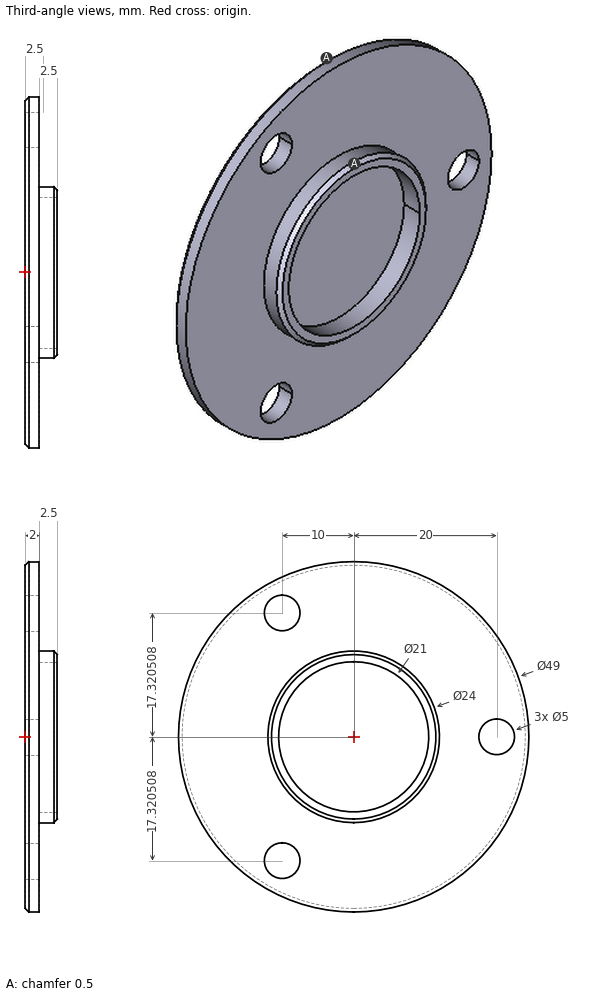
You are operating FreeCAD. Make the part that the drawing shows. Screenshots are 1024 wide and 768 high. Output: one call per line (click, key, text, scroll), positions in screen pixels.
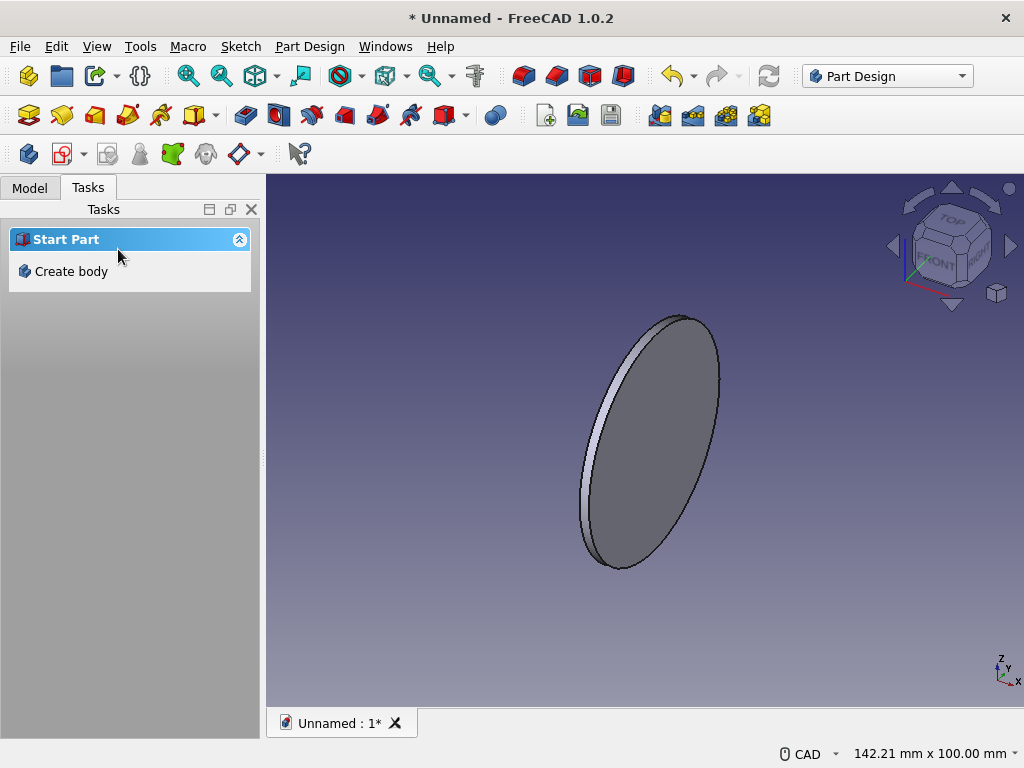
click(654, 443)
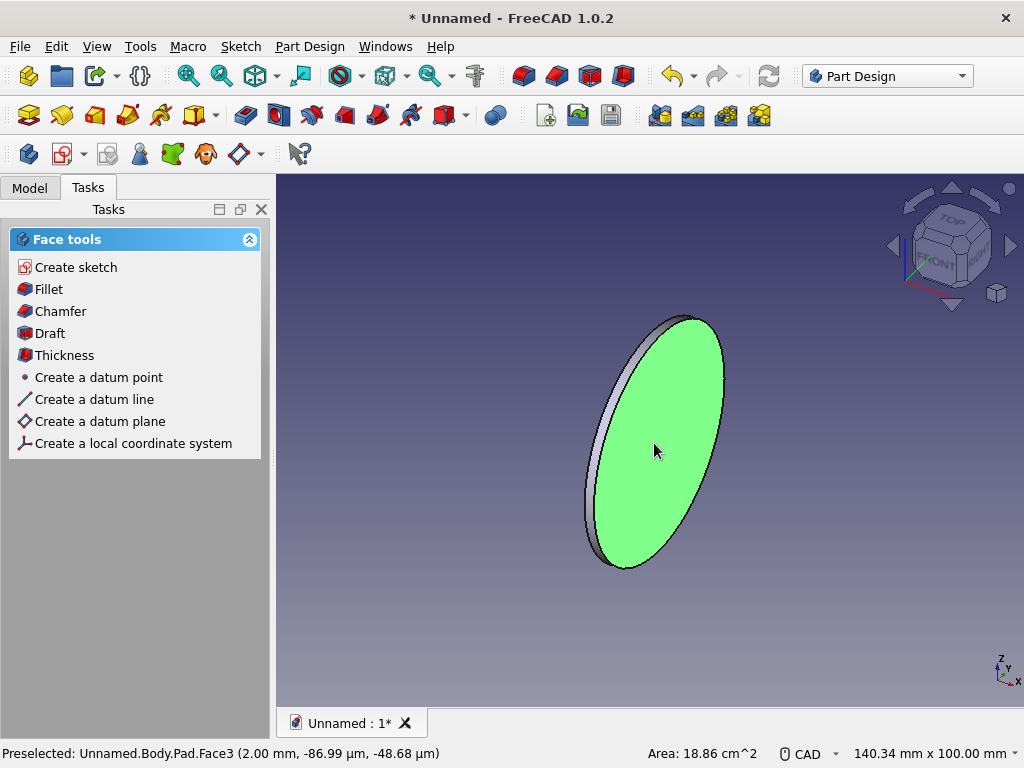
click(62, 154)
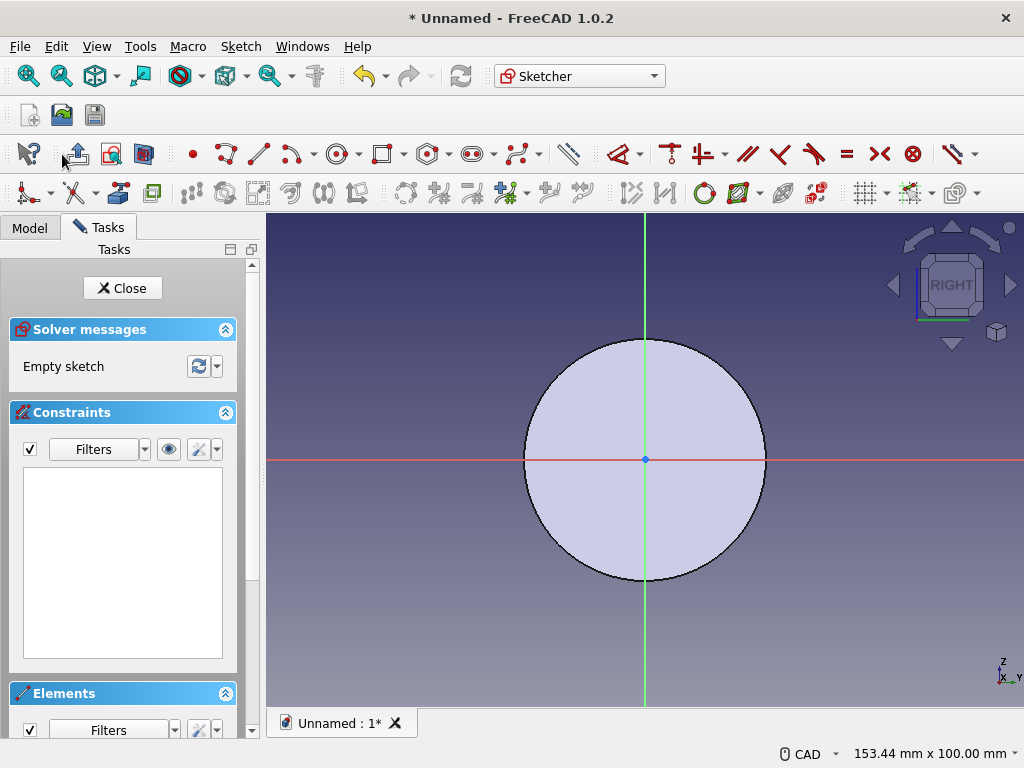
scroll(685, 460, up, 5)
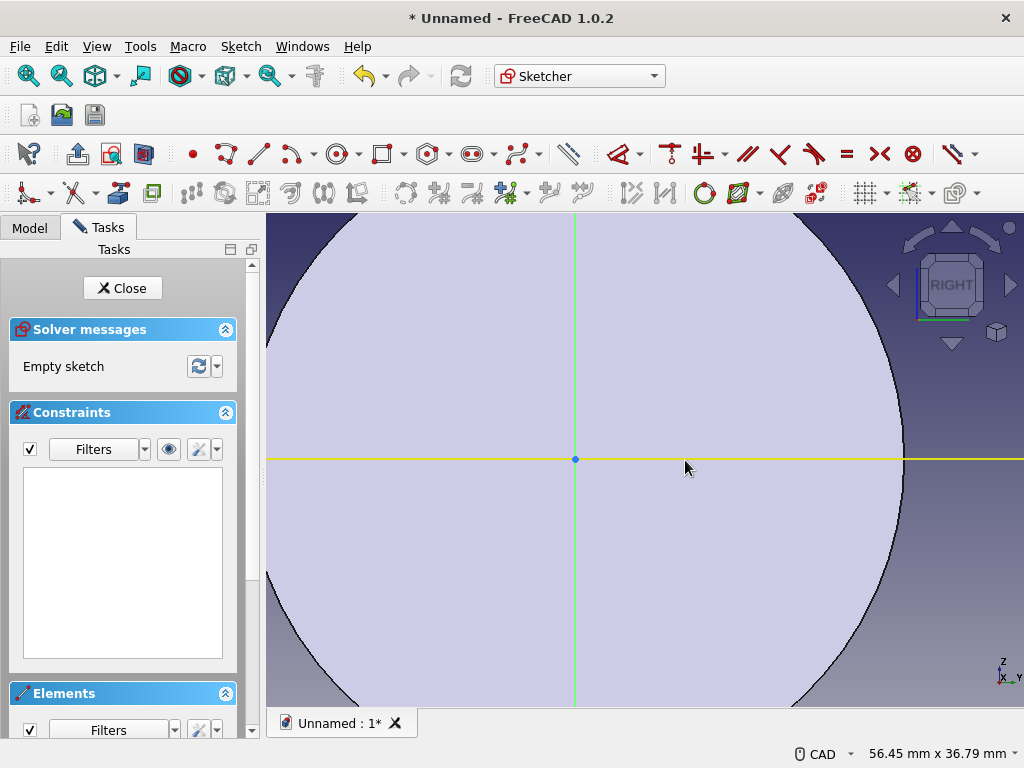
click(336, 154)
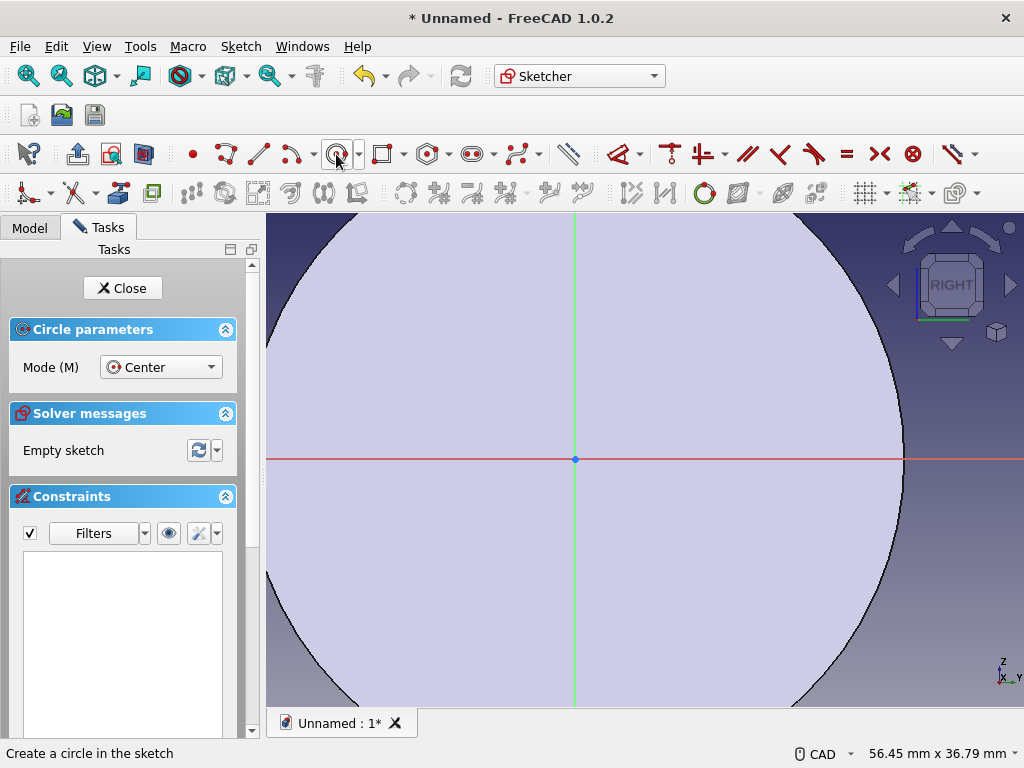
click(575, 459)
click(689, 345)
key(Escape)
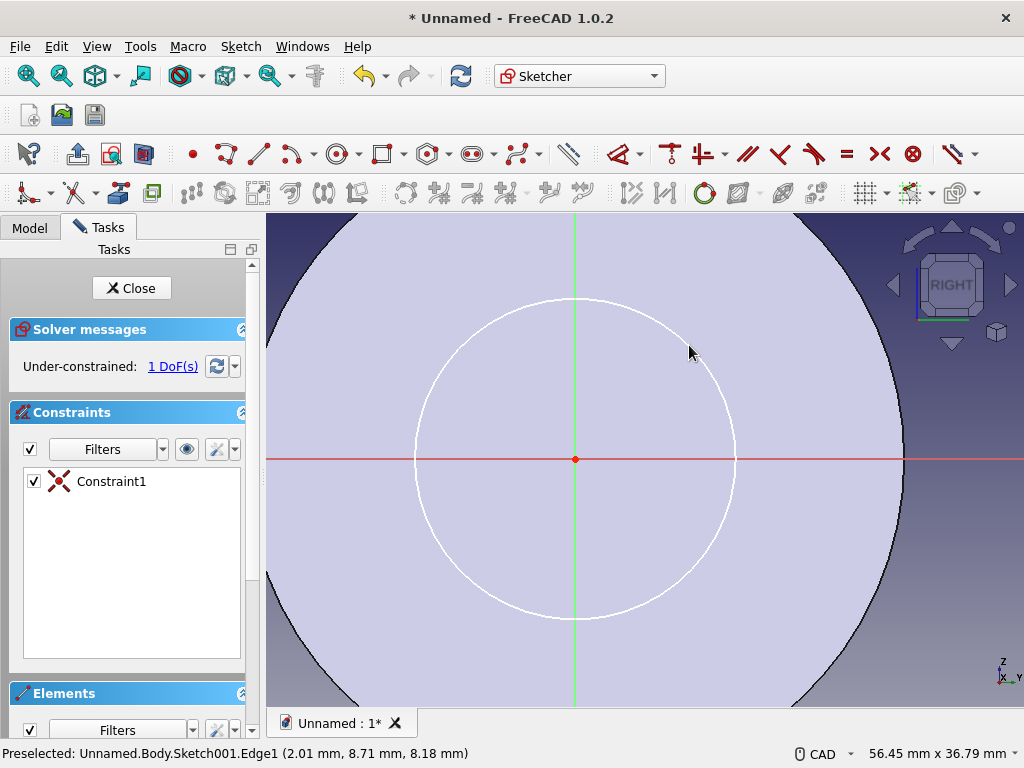
click(618, 154)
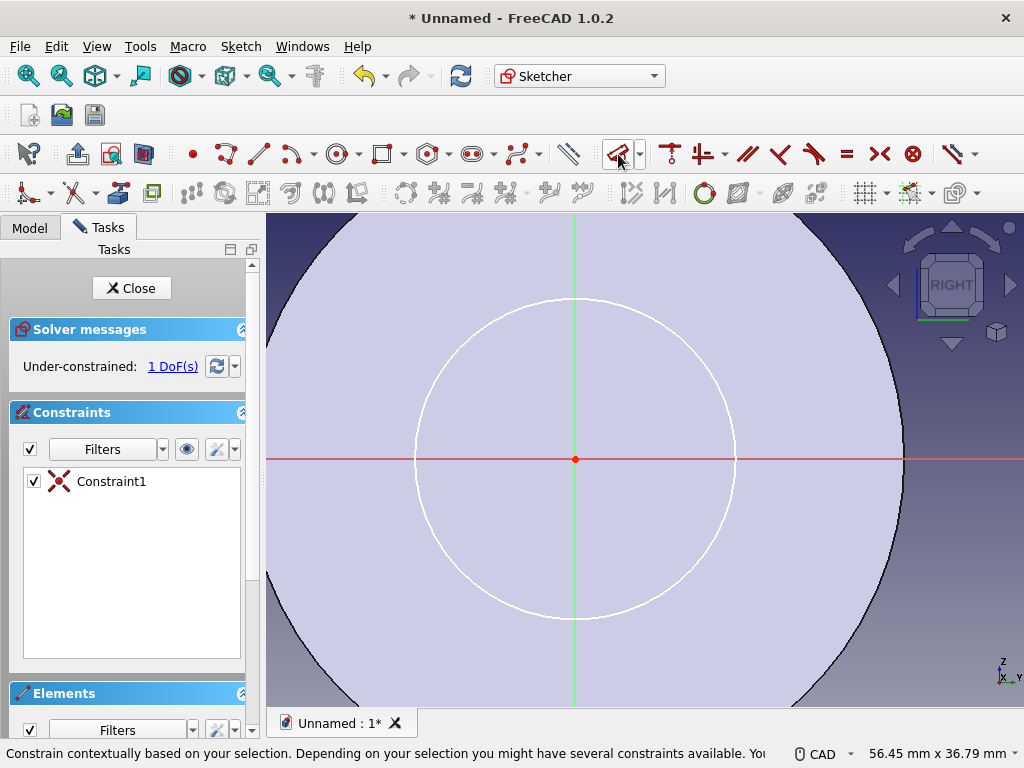
click(688, 345)
click(710, 322)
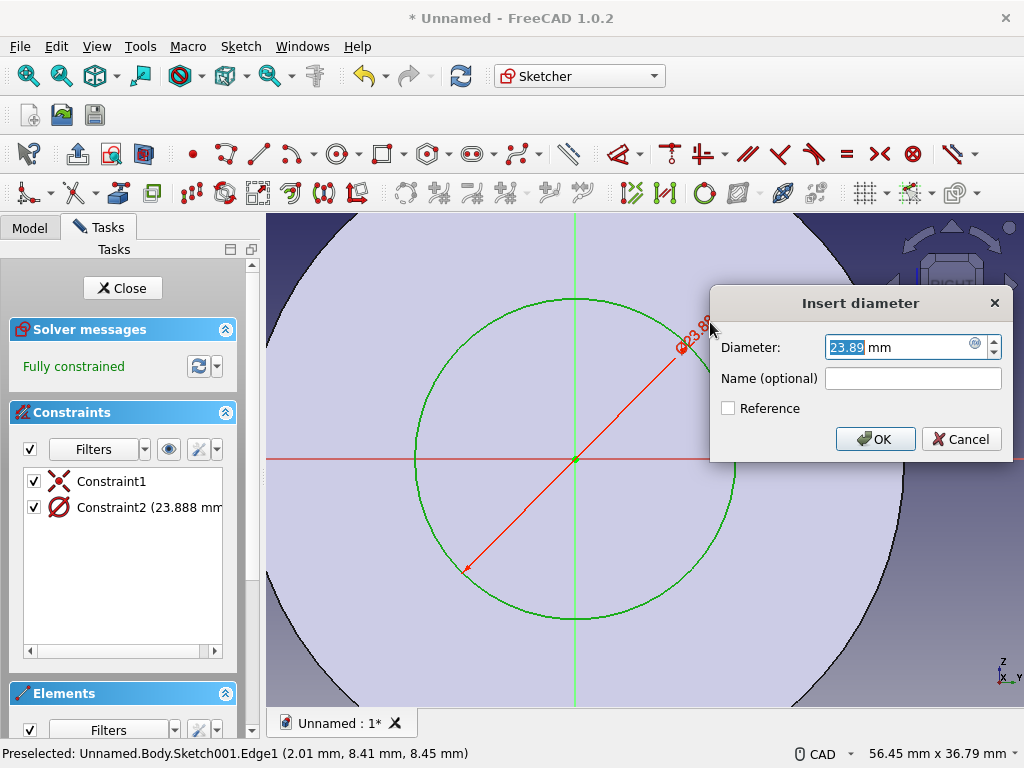
text(24)
key(Return)
key(Escape)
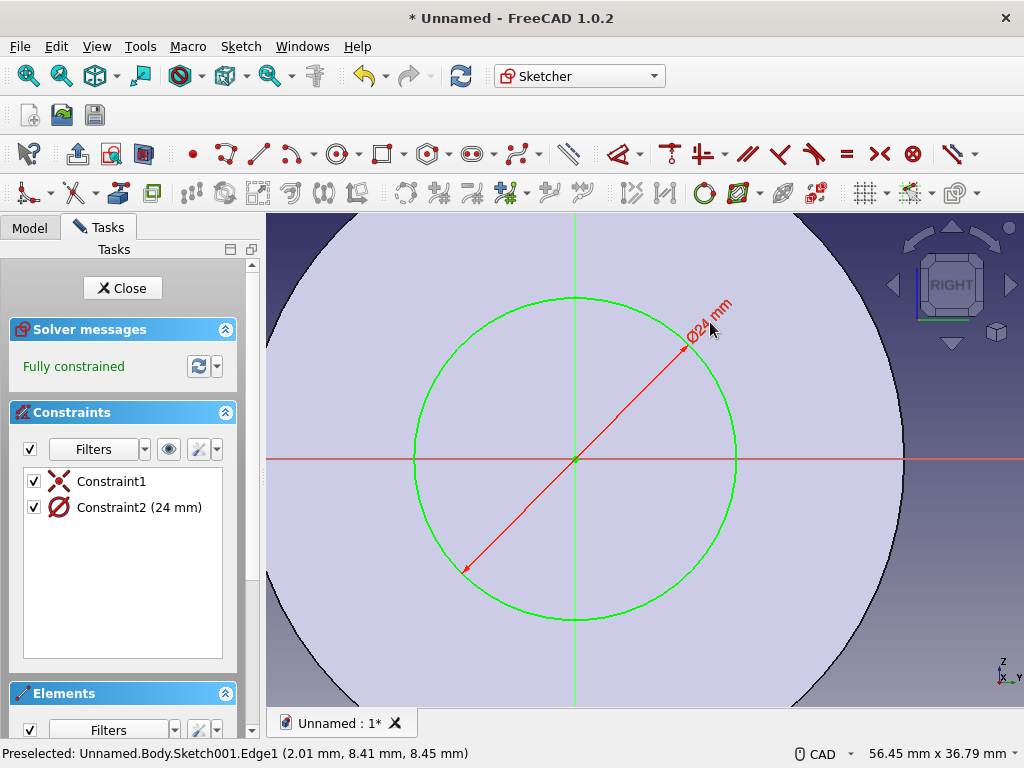
click(123, 288)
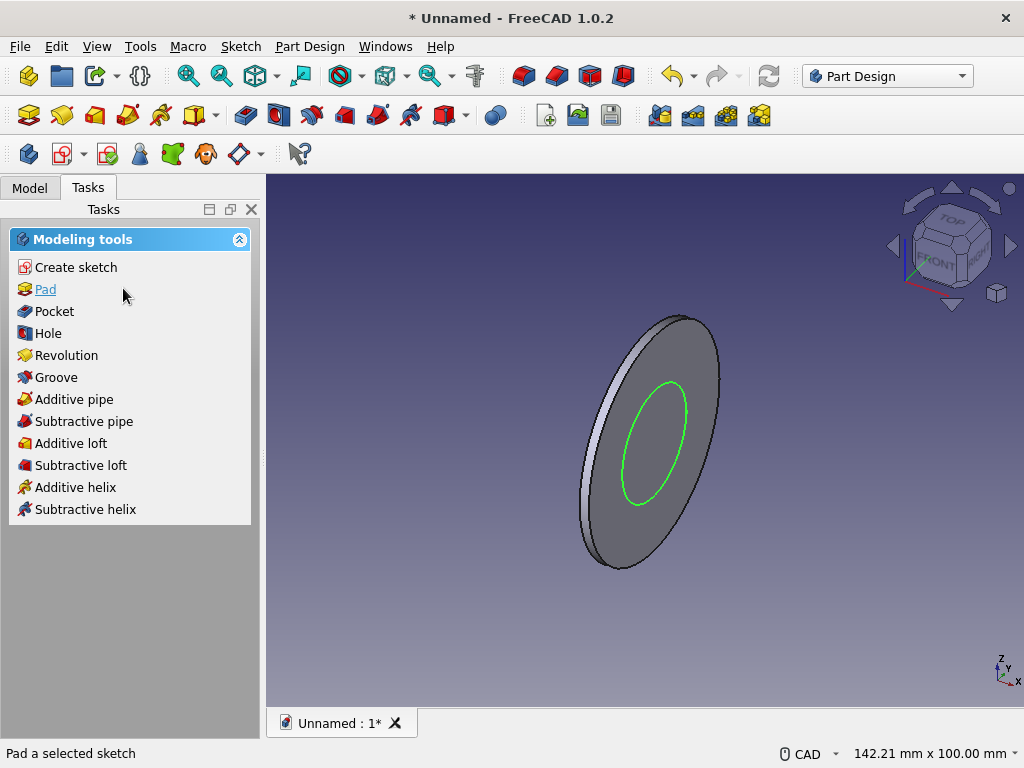
click(29, 116)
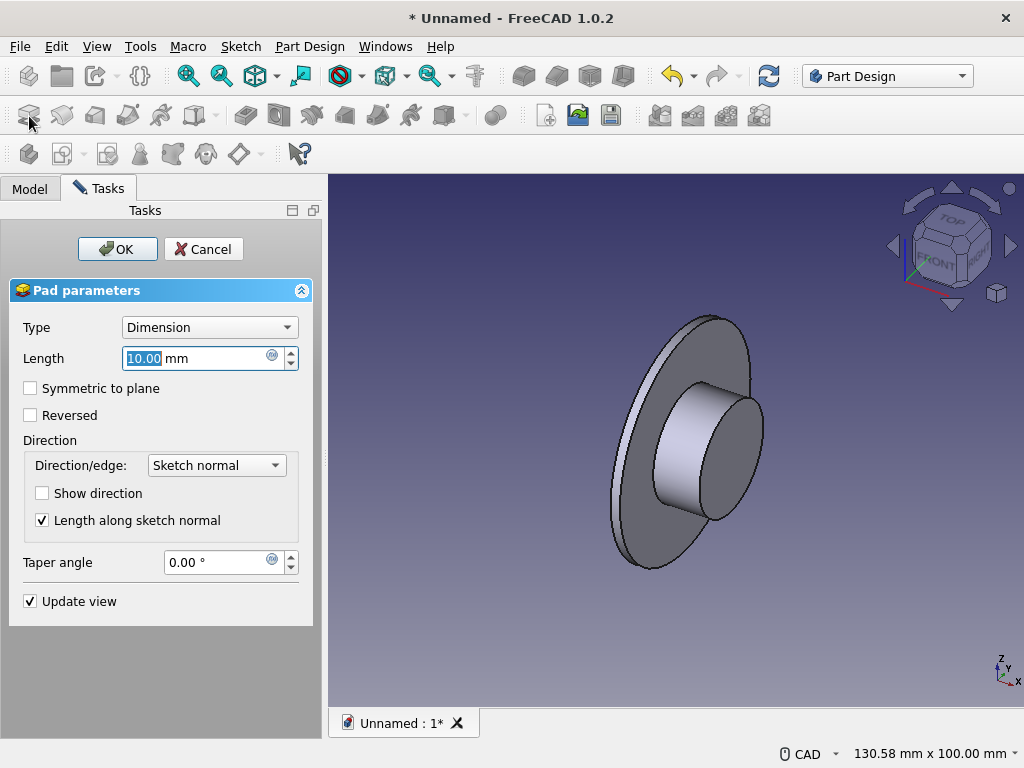
text(2.5)
key(Tab)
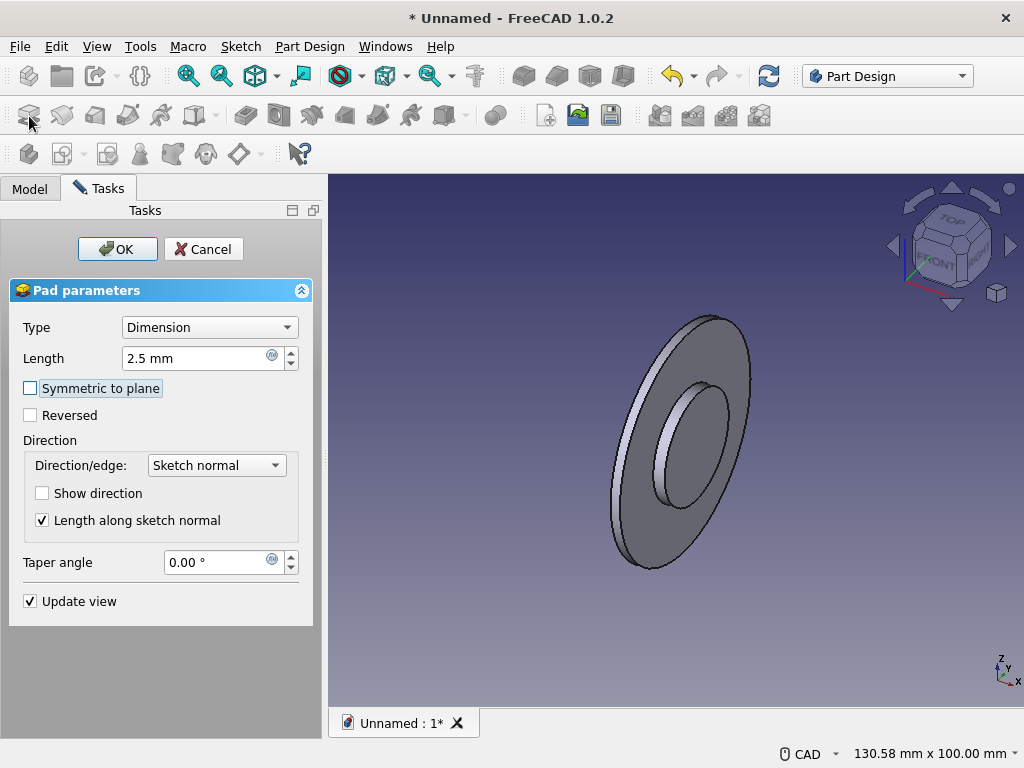
click(118, 249)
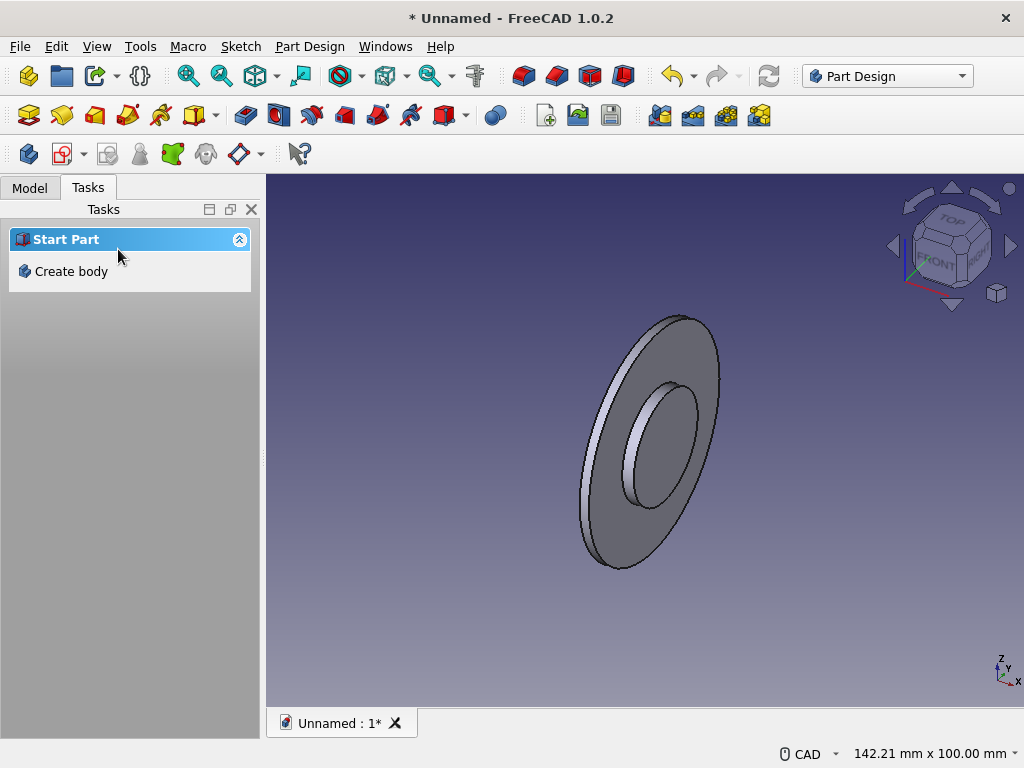
click(666, 446)